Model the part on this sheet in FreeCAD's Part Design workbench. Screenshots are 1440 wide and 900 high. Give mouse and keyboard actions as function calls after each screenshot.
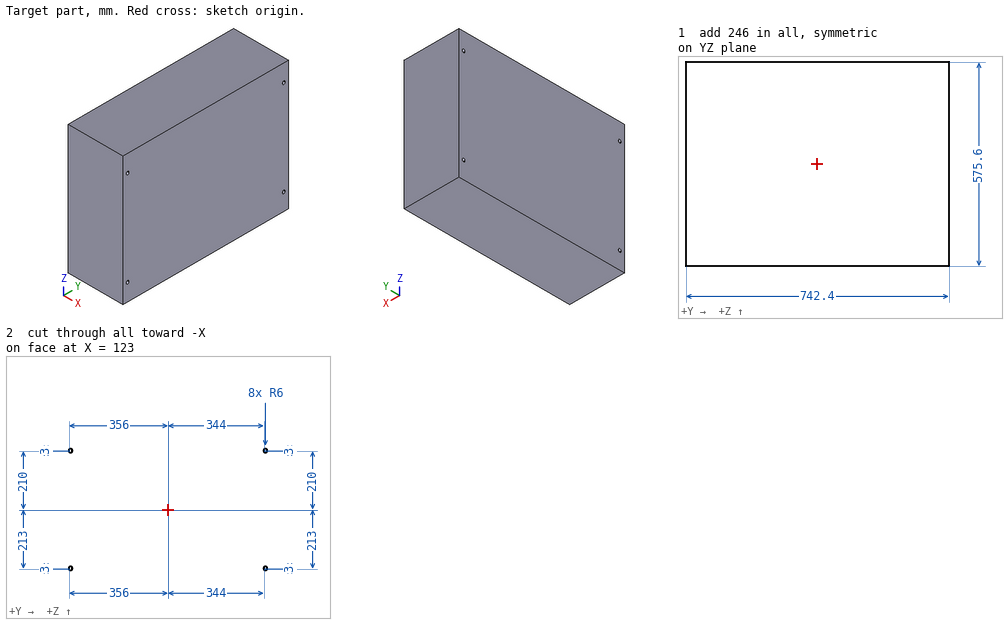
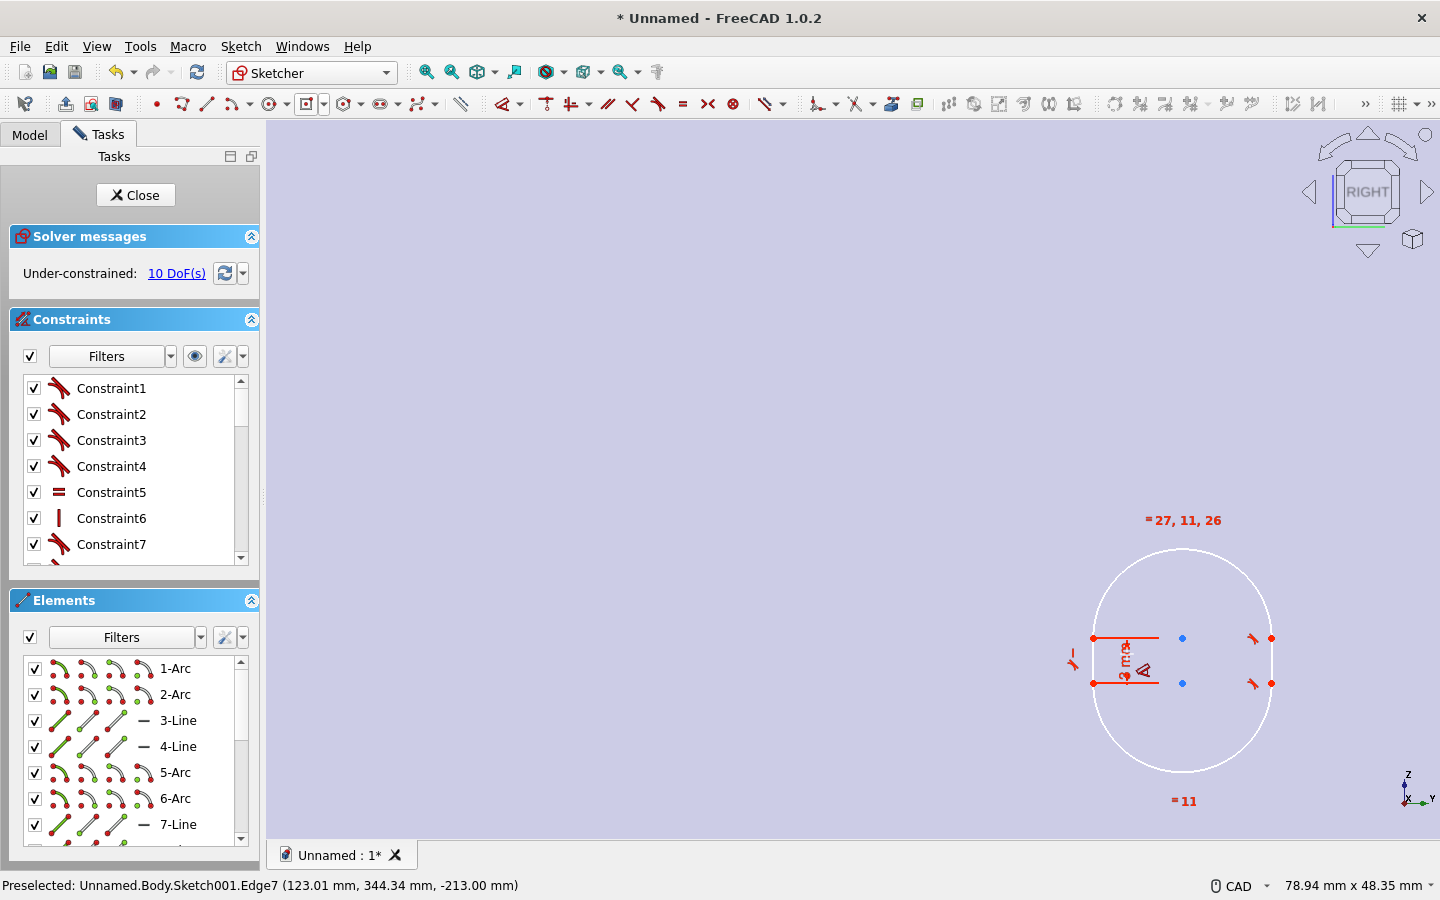
scroll(1096, 672, down, 14)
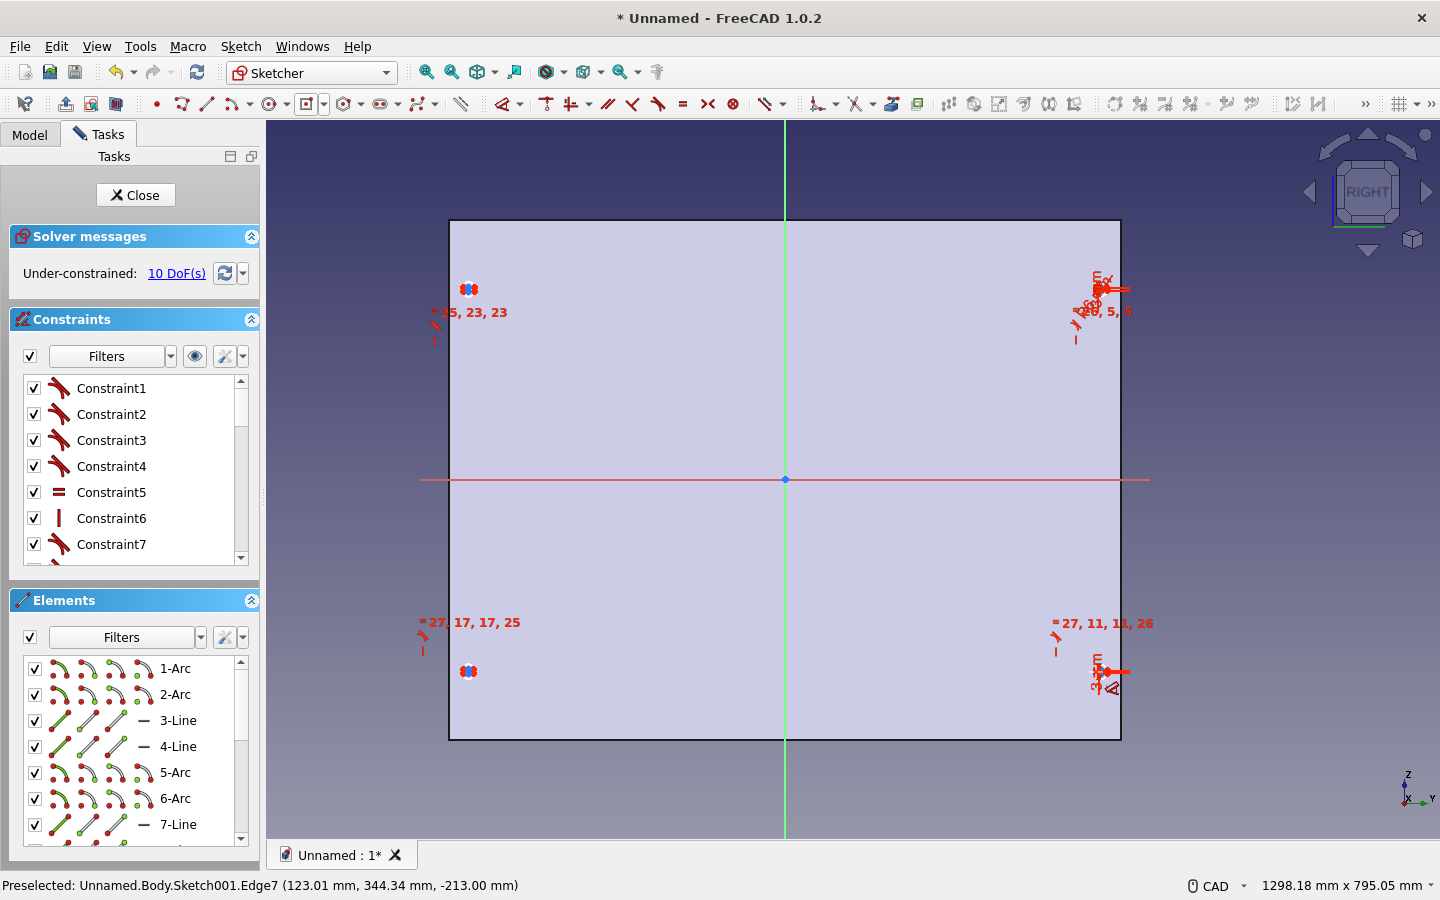
scroll(463, 672, up, 14)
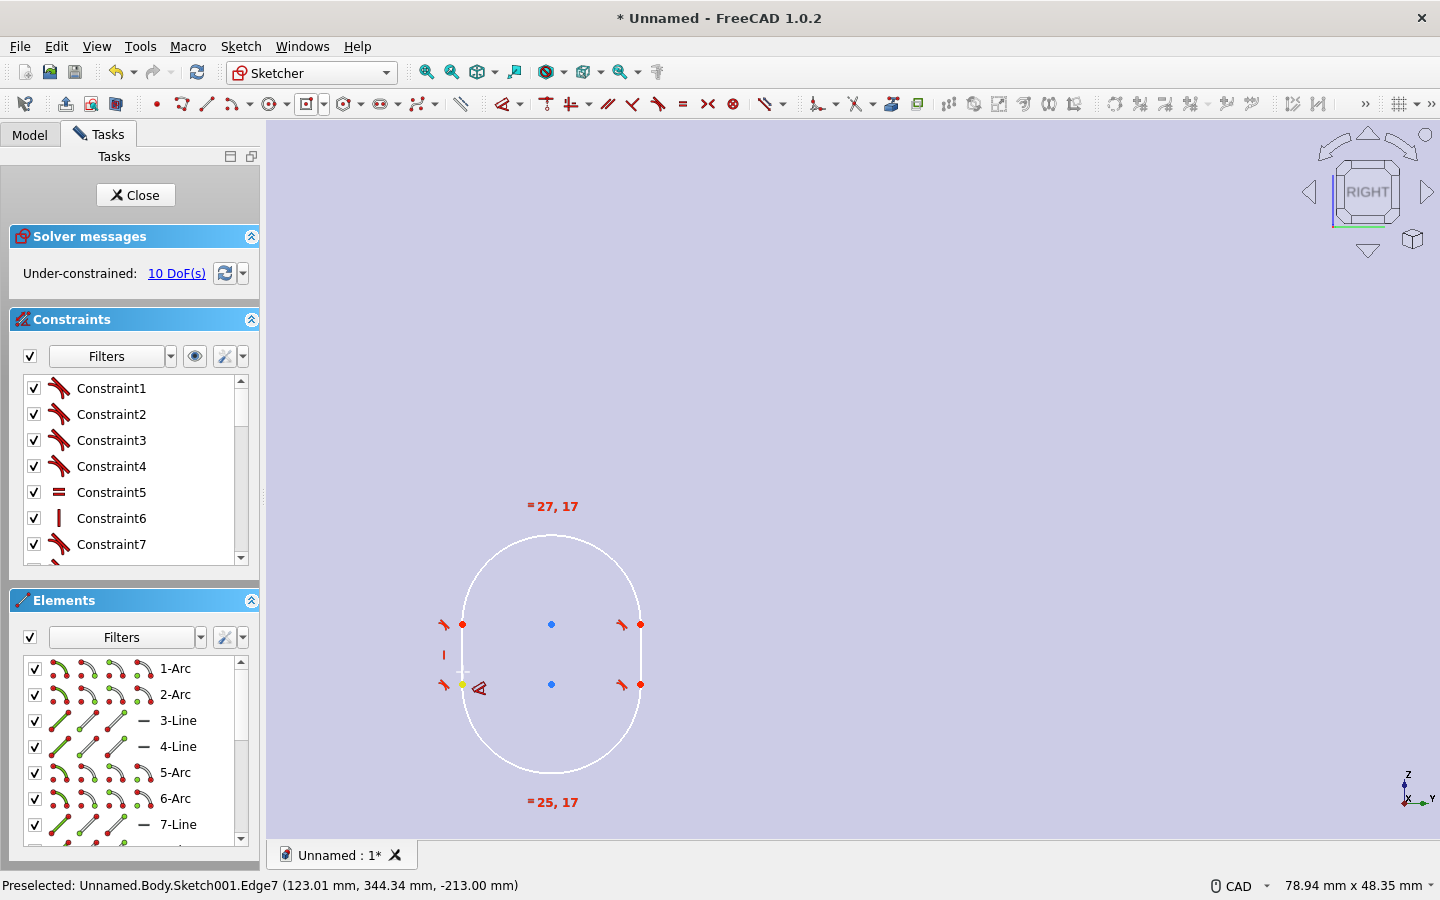
click(462, 666)
click(428, 654)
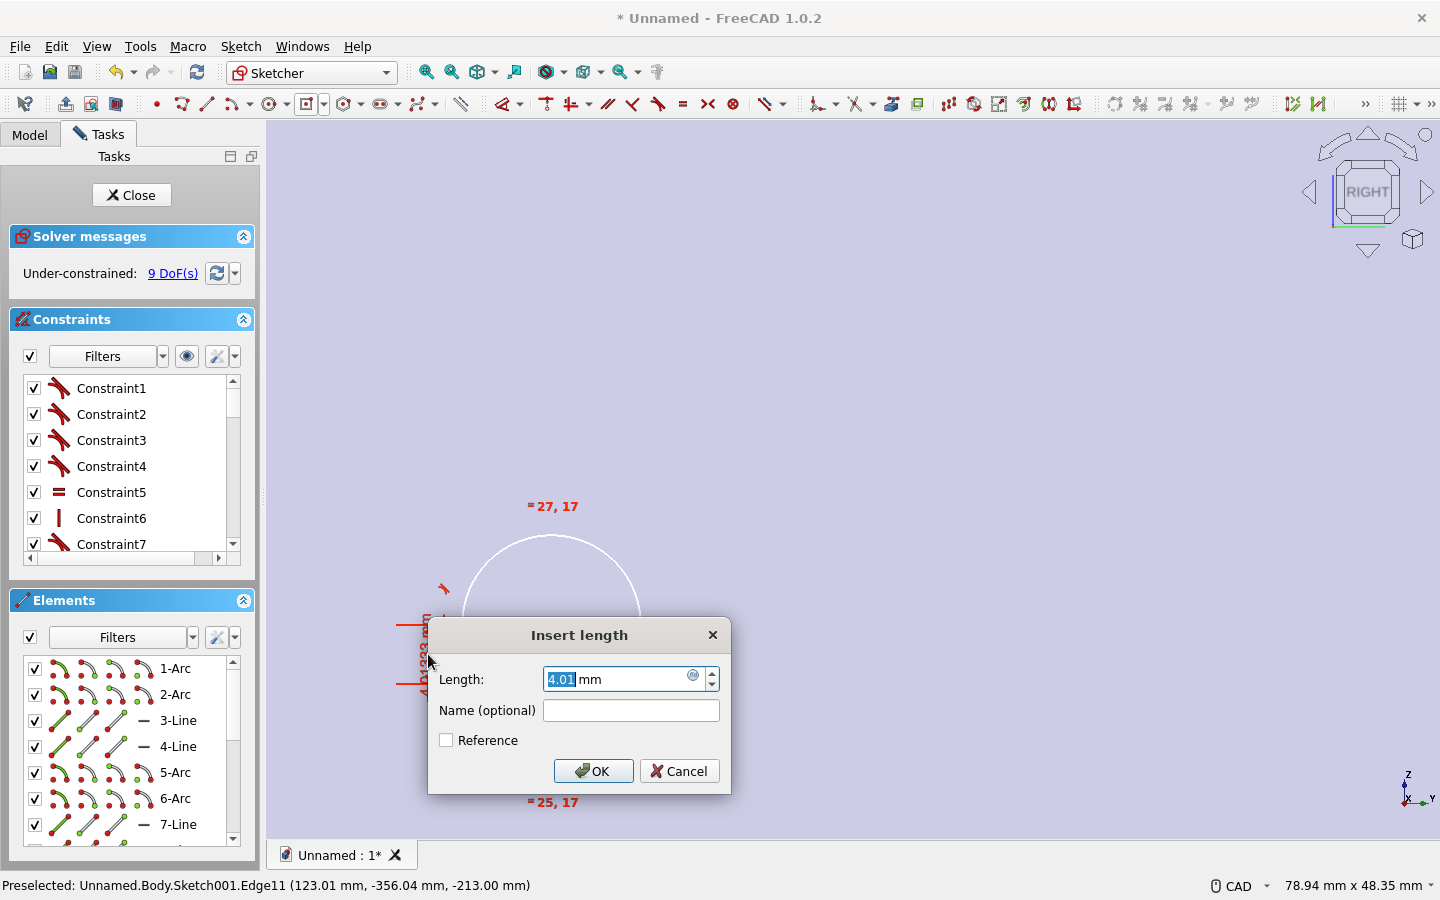
text(3)
key(Return)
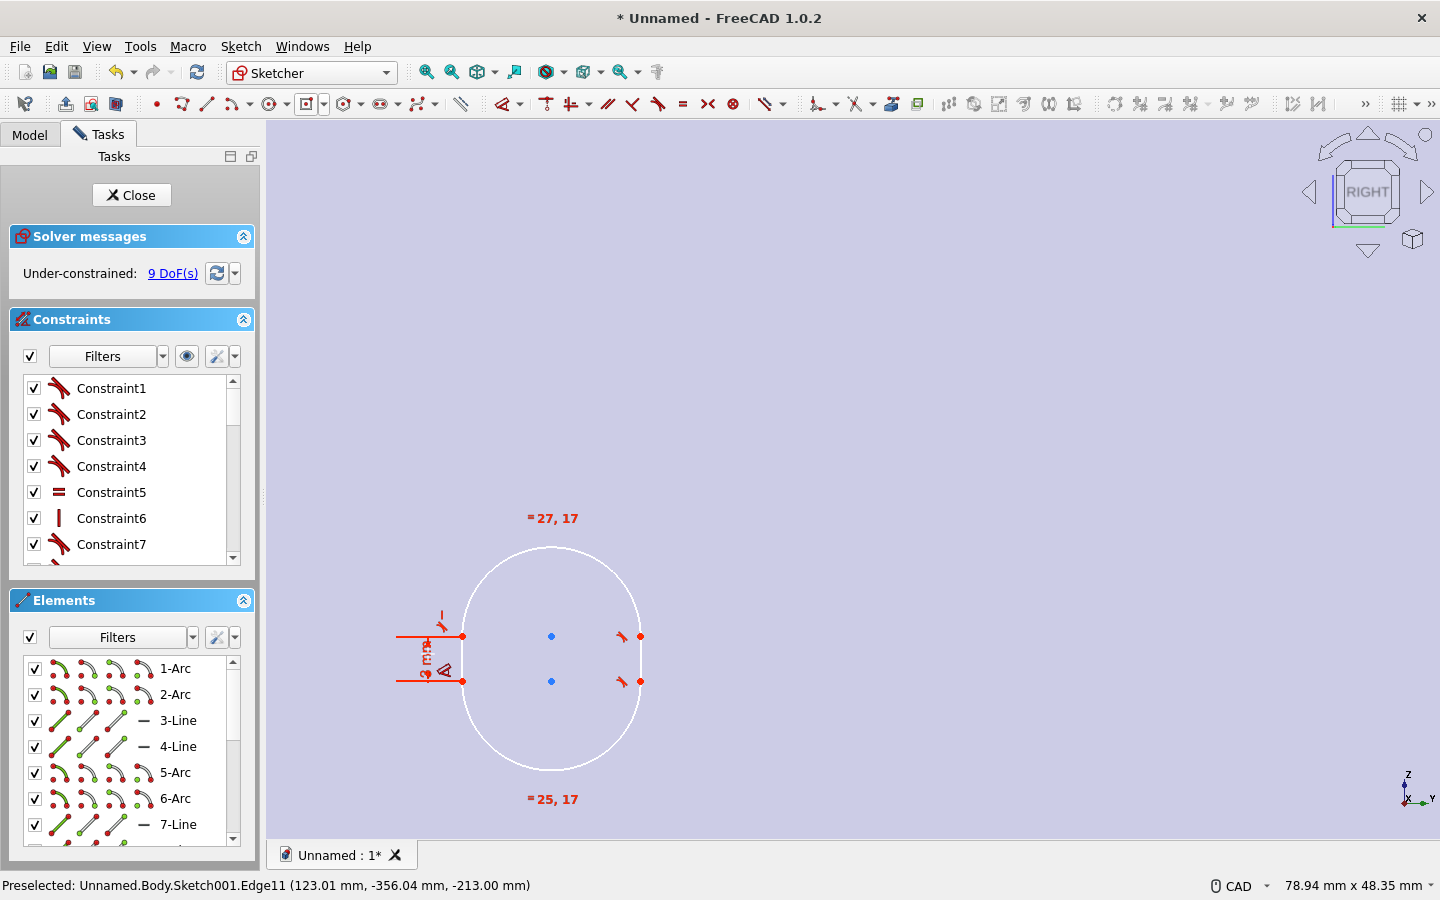
scroll(463, 672, down, 14)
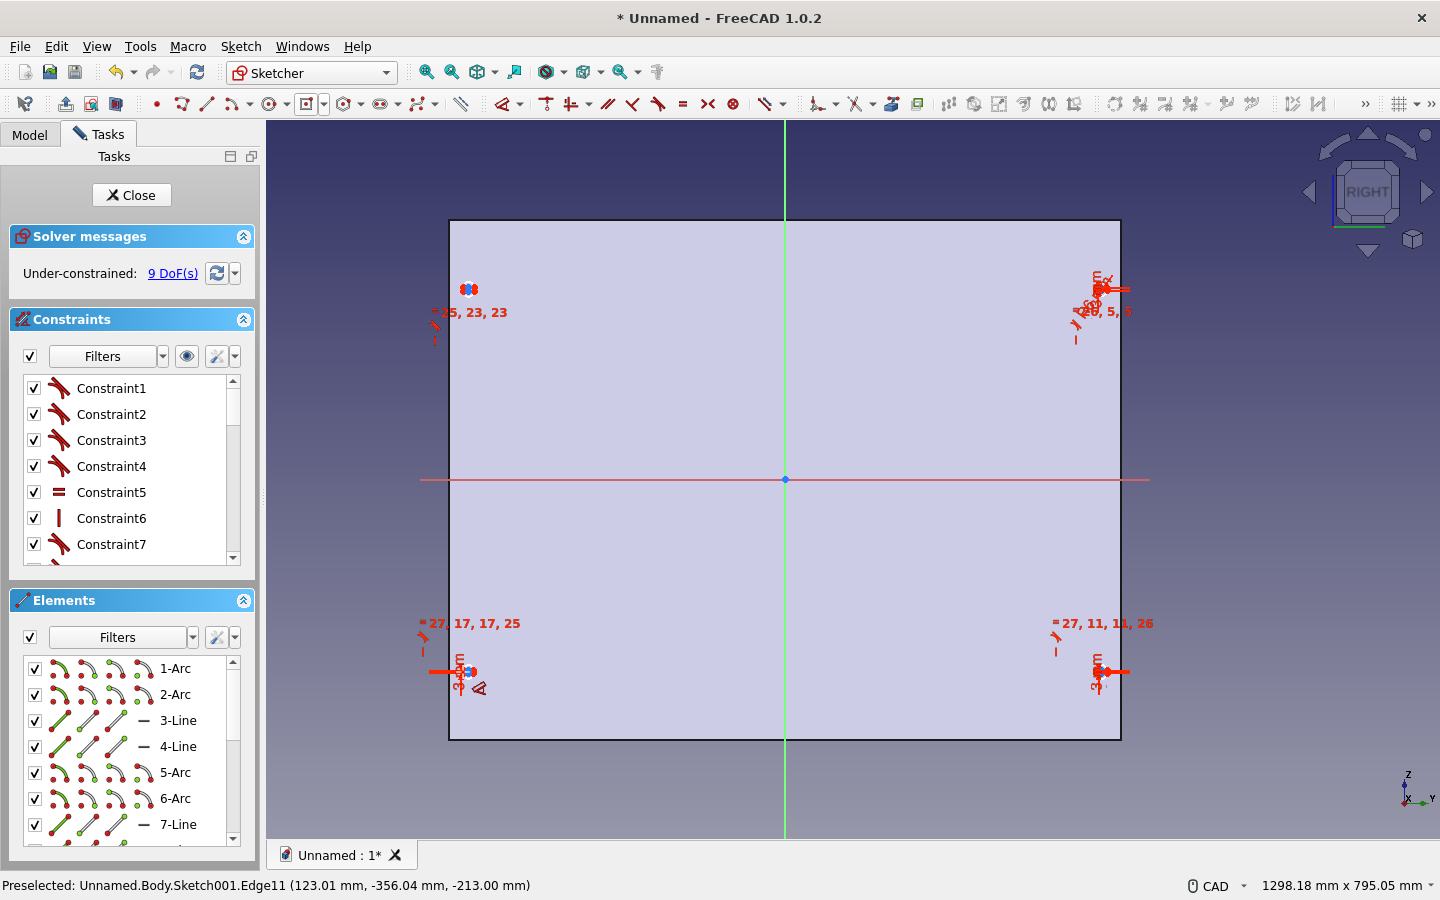
scroll(463, 290, up, 14)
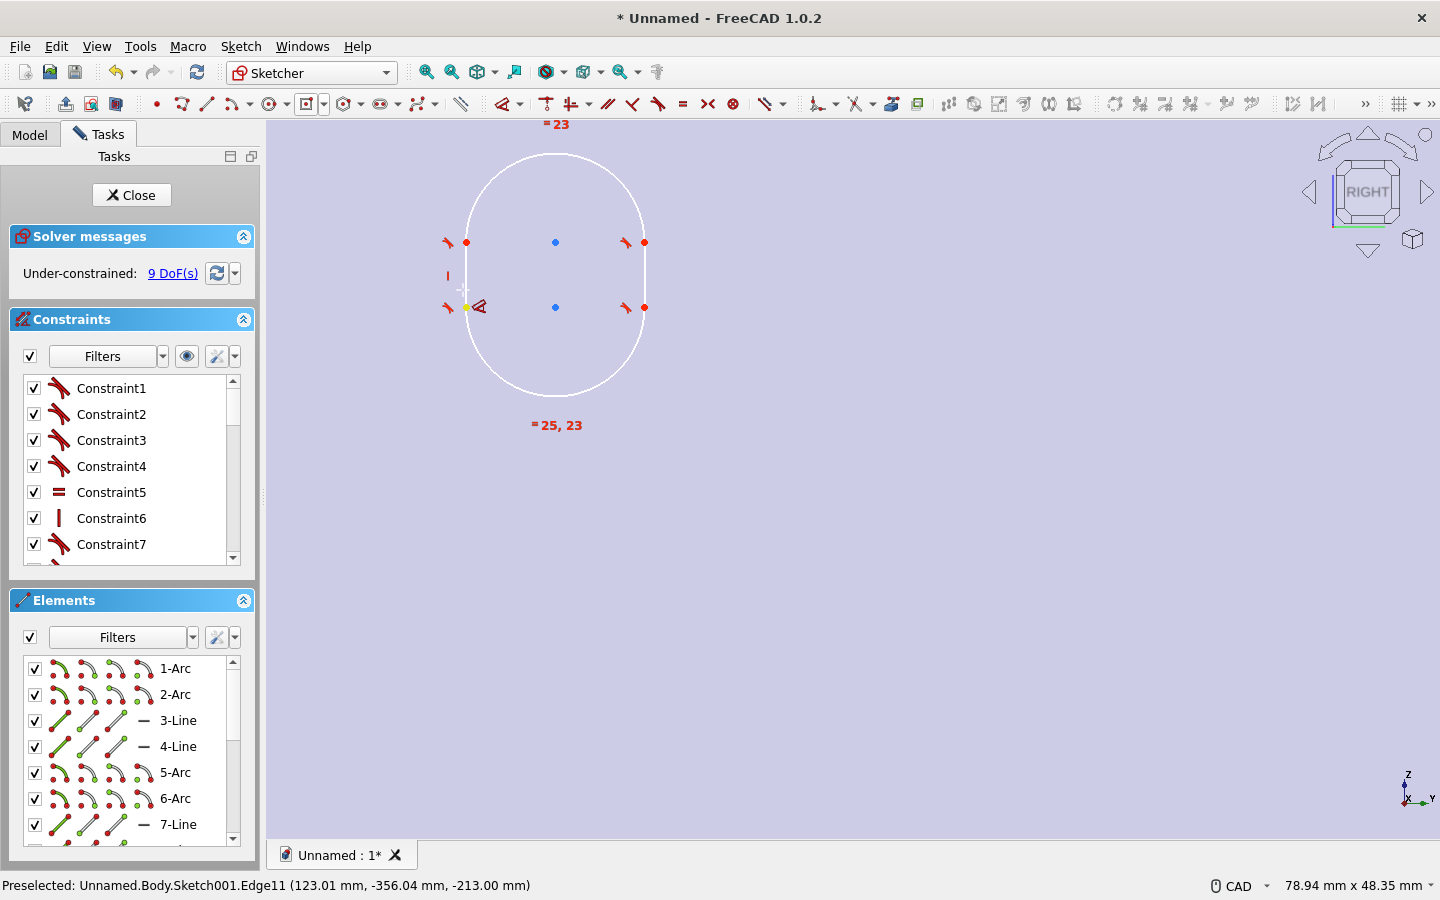
click(466, 288)
click(432, 275)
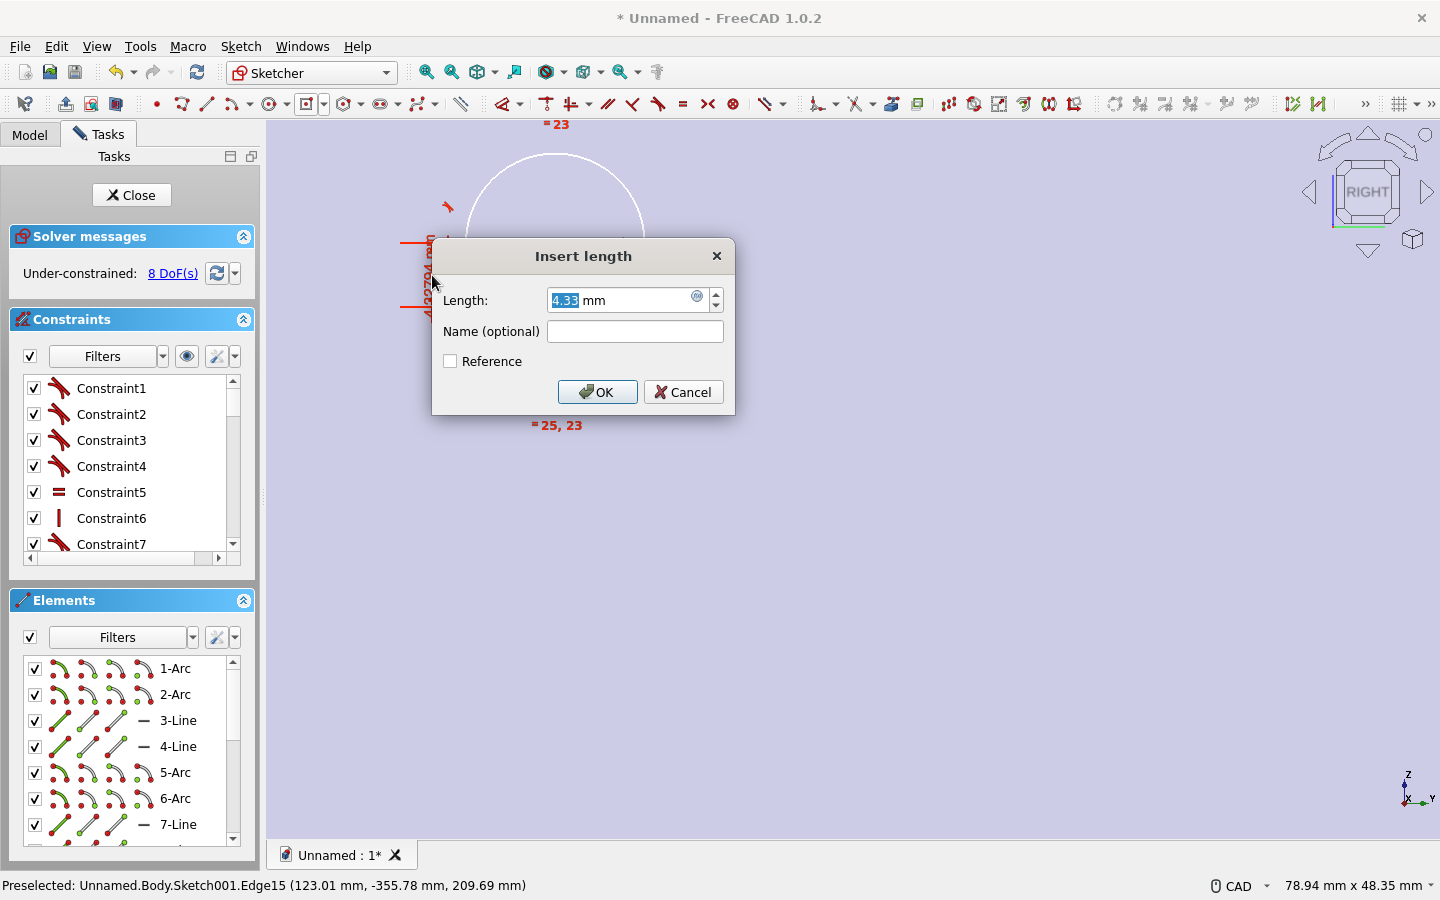
text(3)
key(Return)